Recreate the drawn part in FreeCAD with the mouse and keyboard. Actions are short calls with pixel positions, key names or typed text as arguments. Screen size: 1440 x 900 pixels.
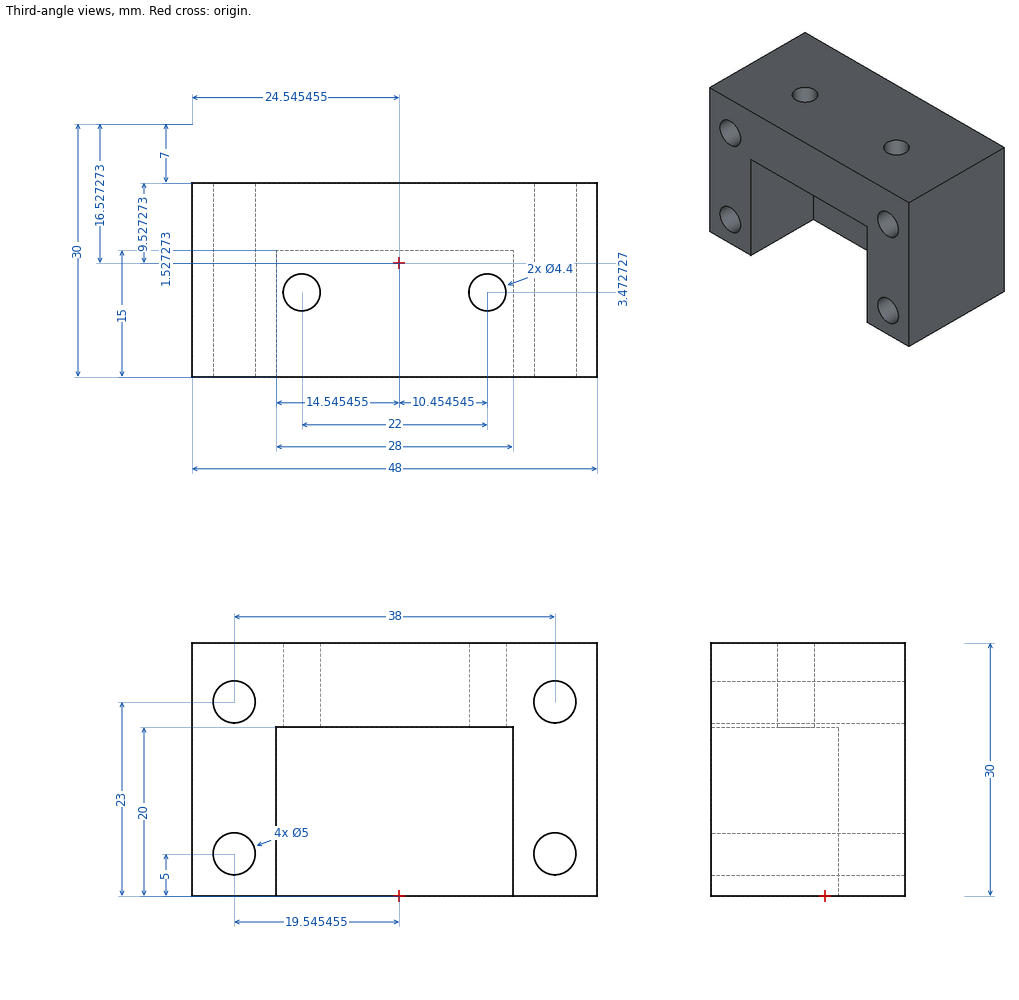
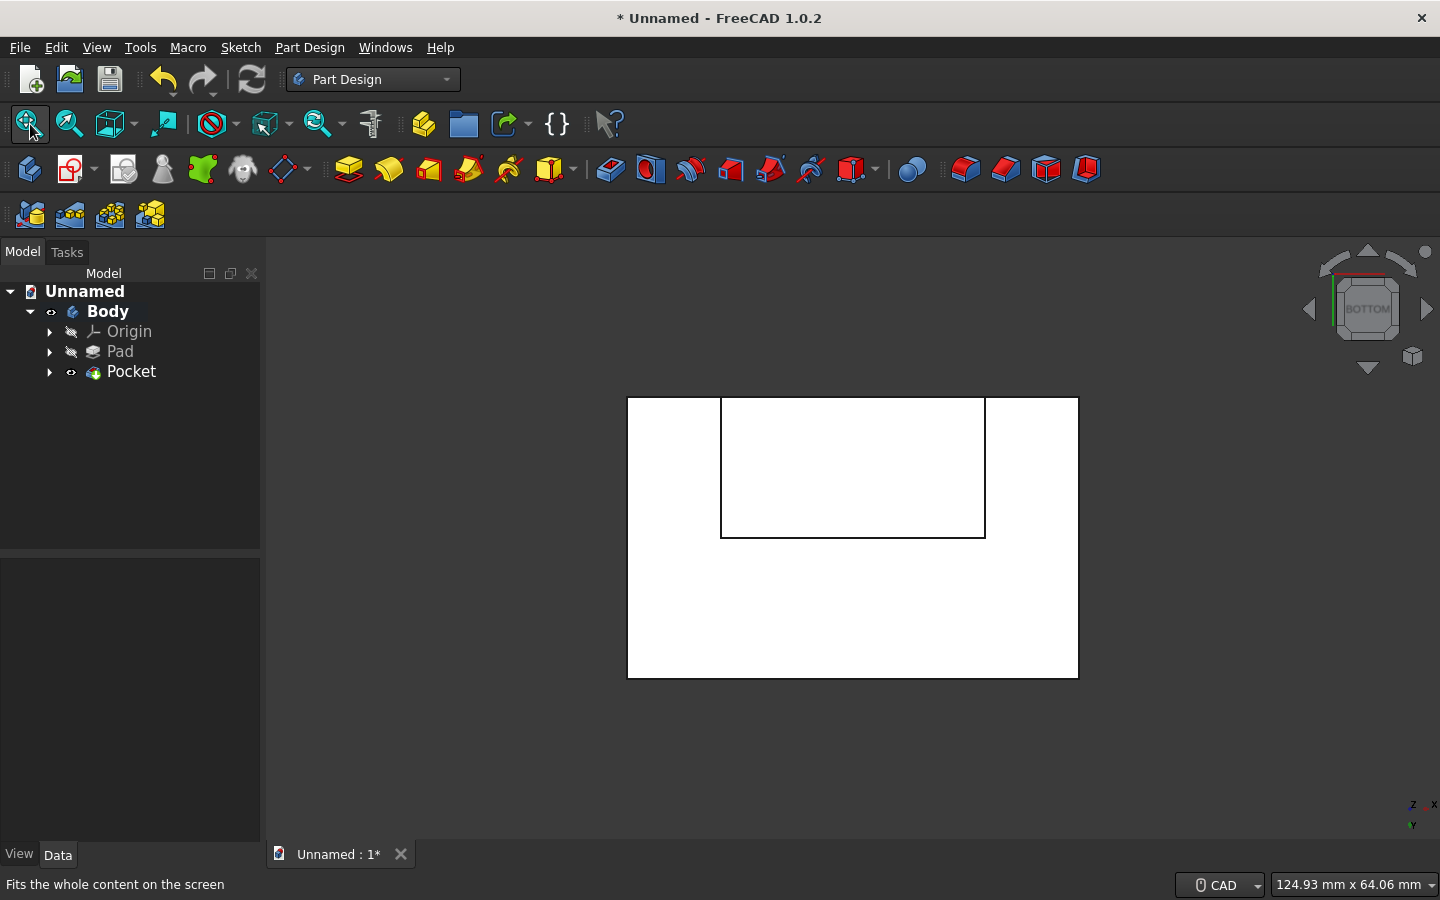
click(891, 467)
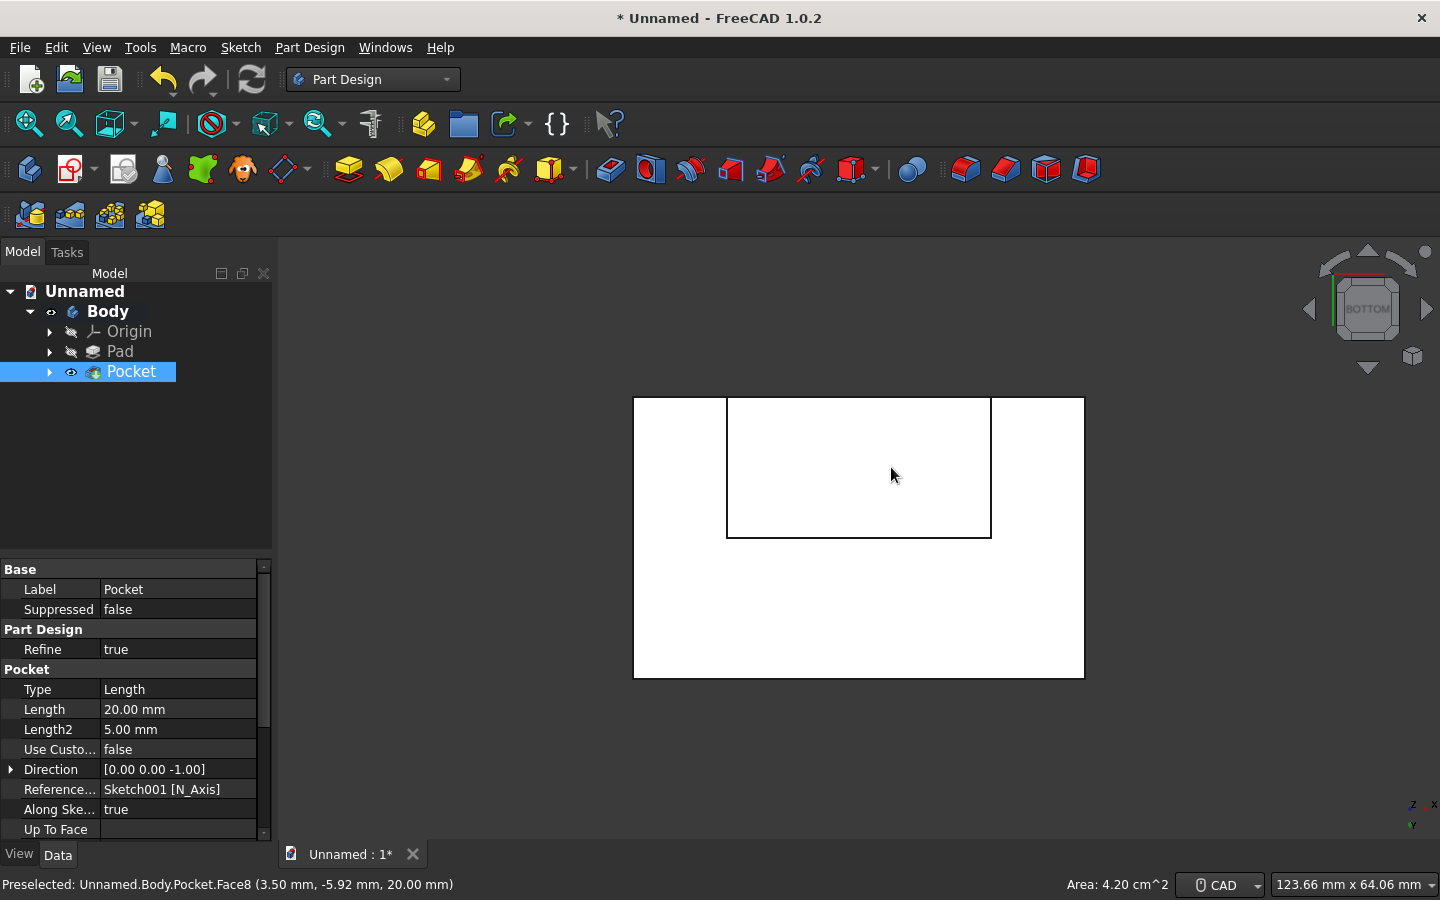
click(70, 170)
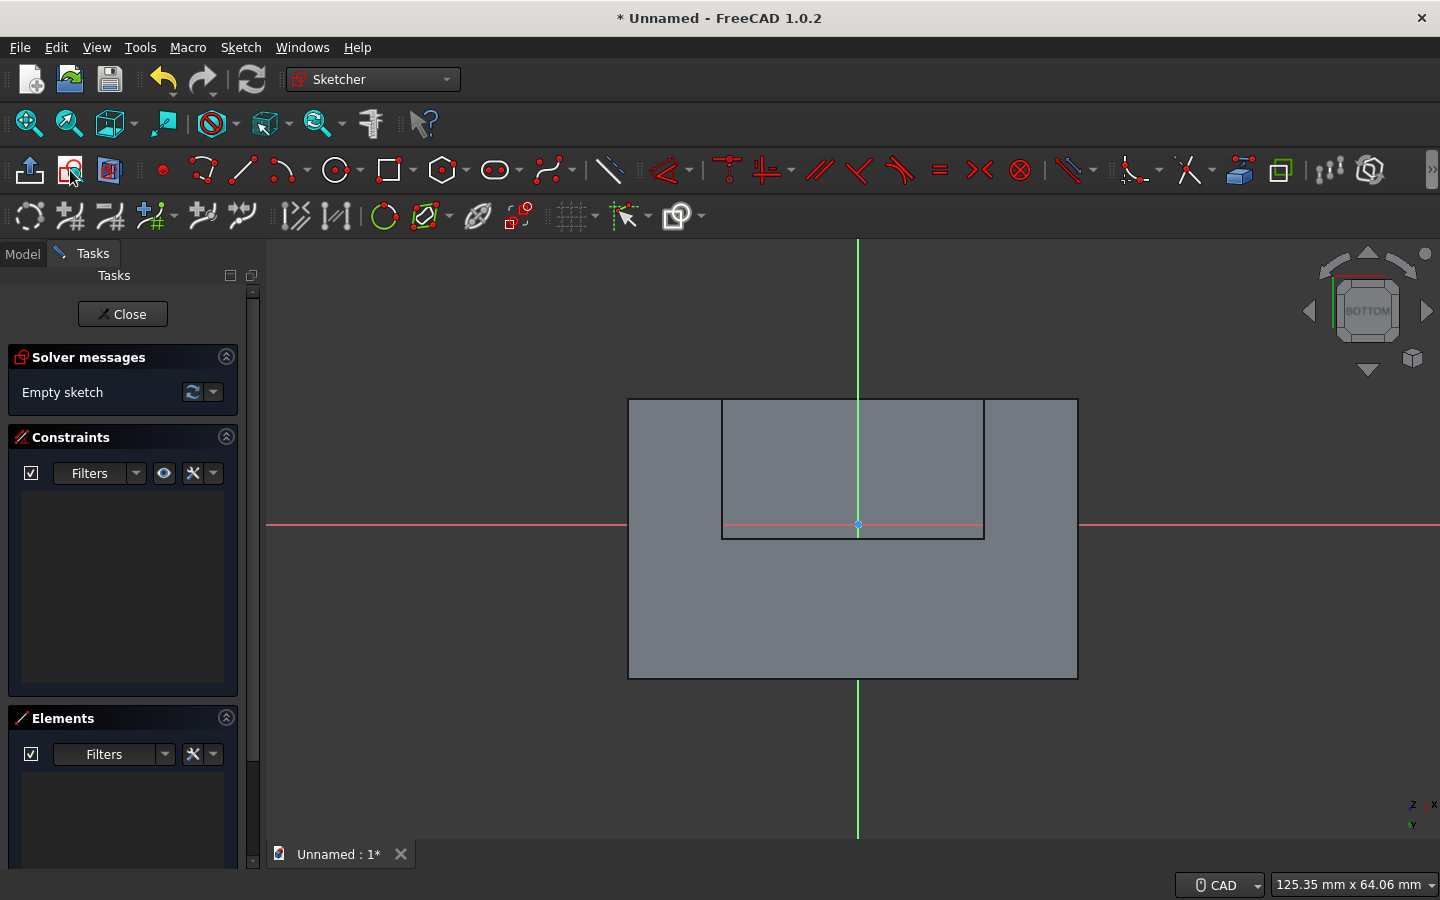
scroll(893, 474, up, 5)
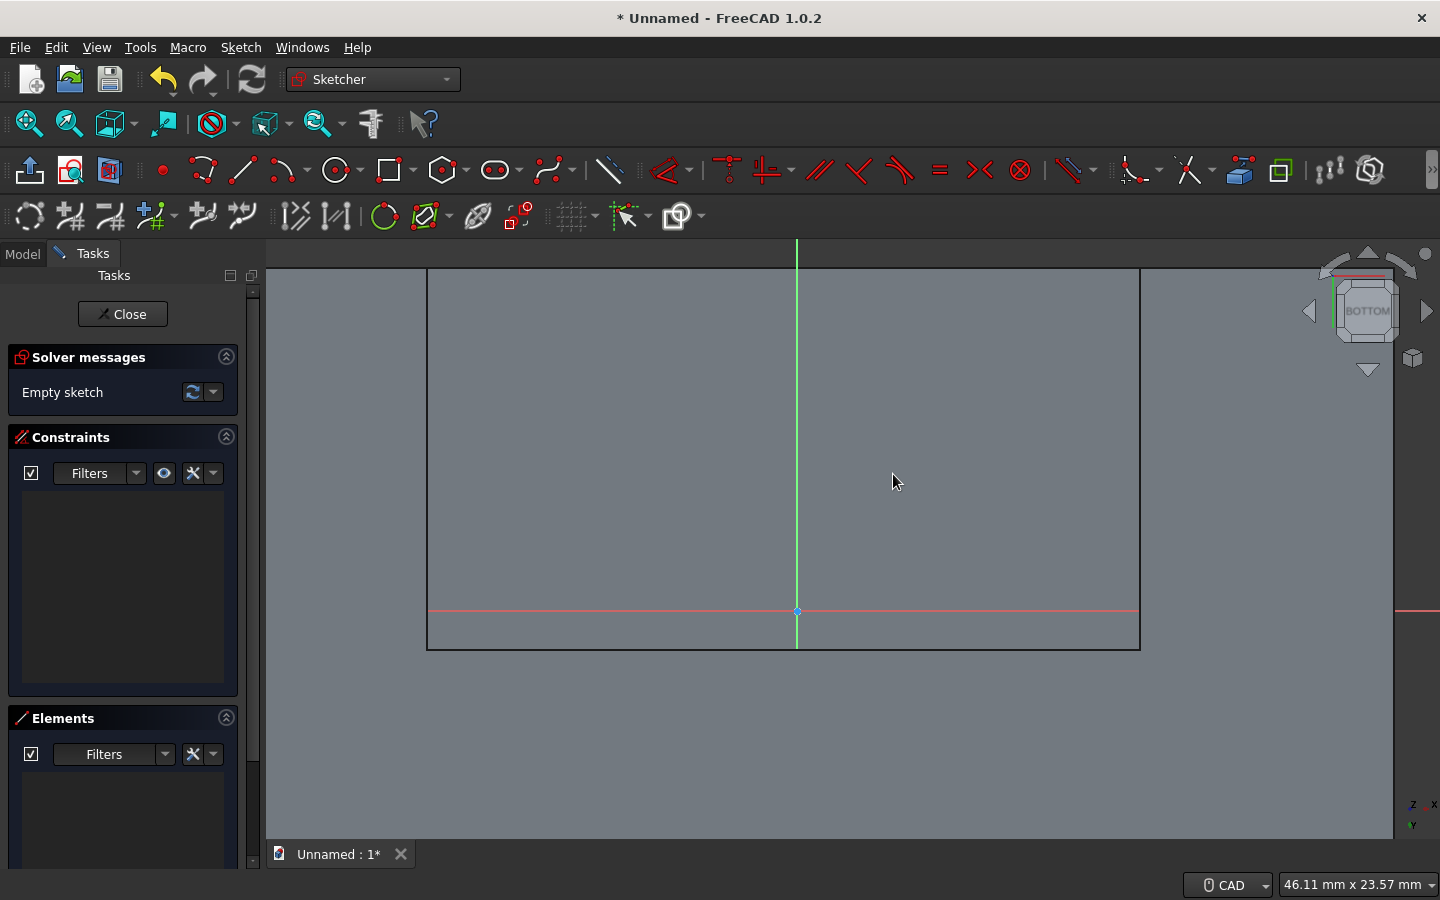
click(336, 170)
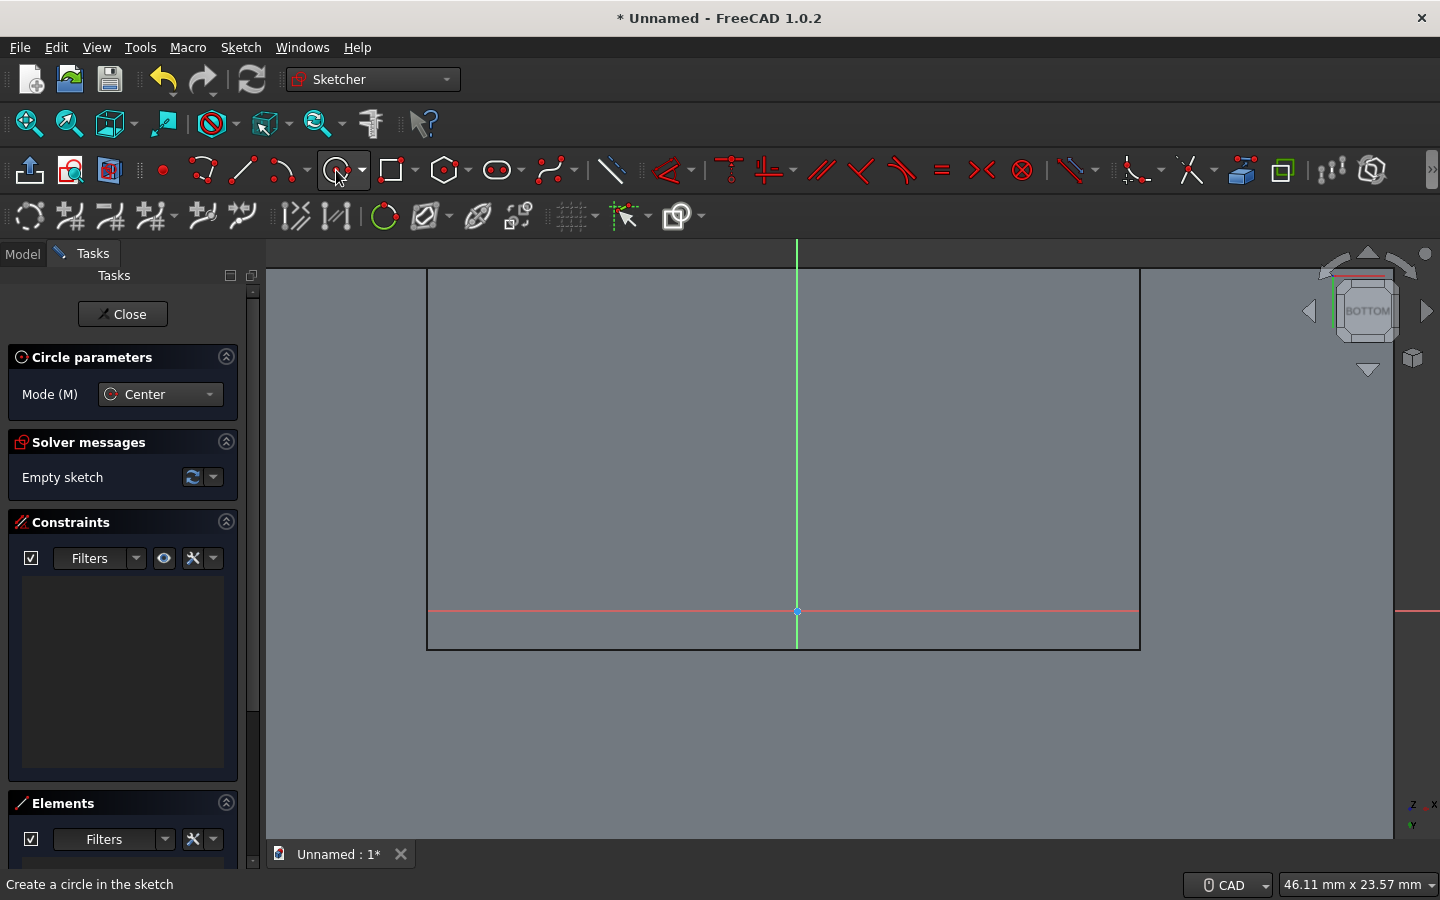
click(1063, 523)
click(1103, 483)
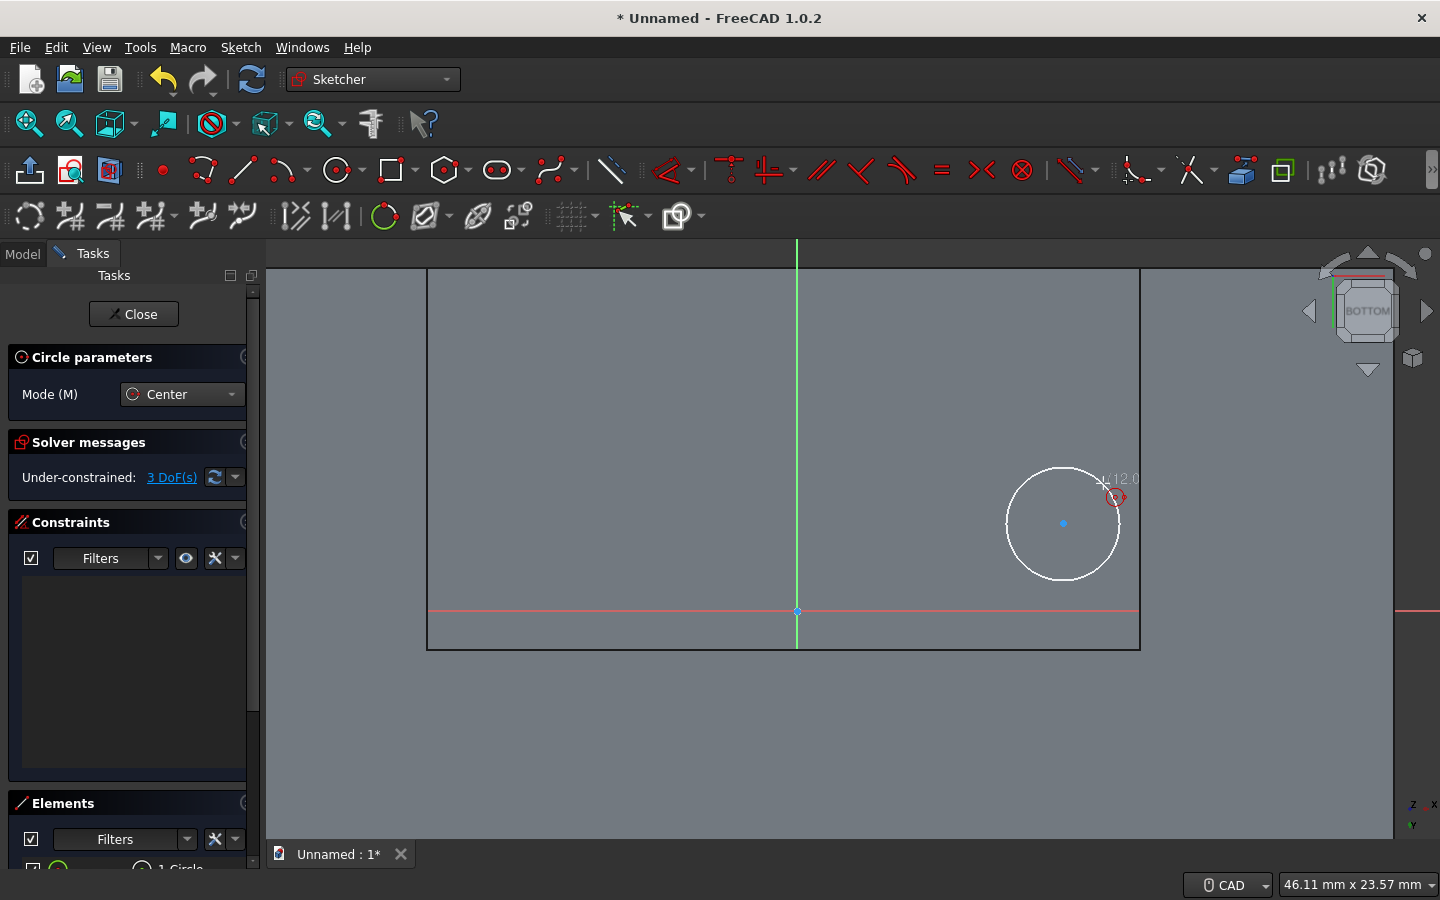
click(503, 523)
click(543, 483)
key(Escape)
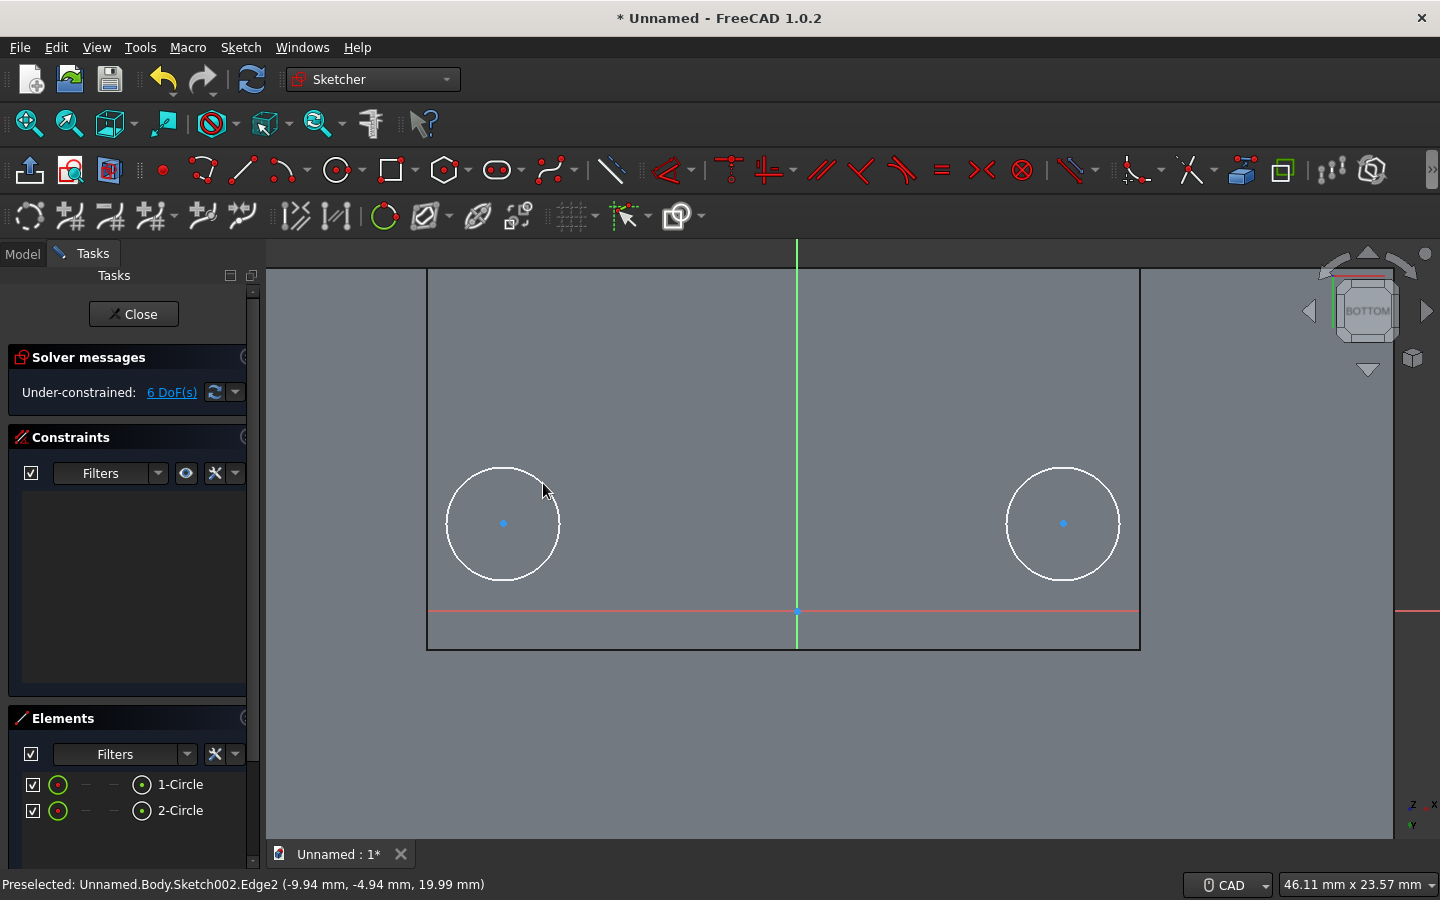
click(1103, 484)